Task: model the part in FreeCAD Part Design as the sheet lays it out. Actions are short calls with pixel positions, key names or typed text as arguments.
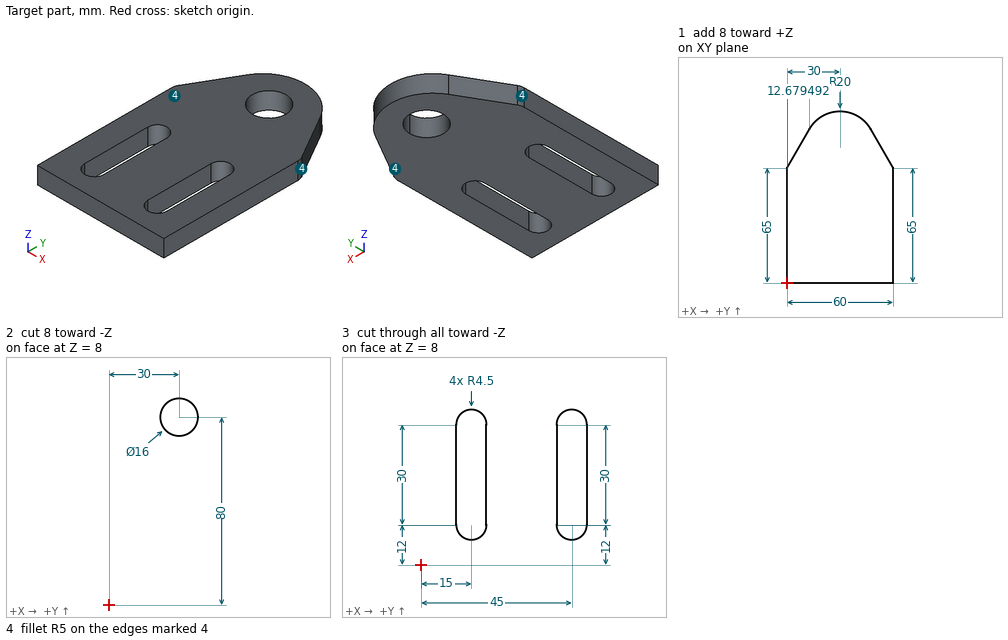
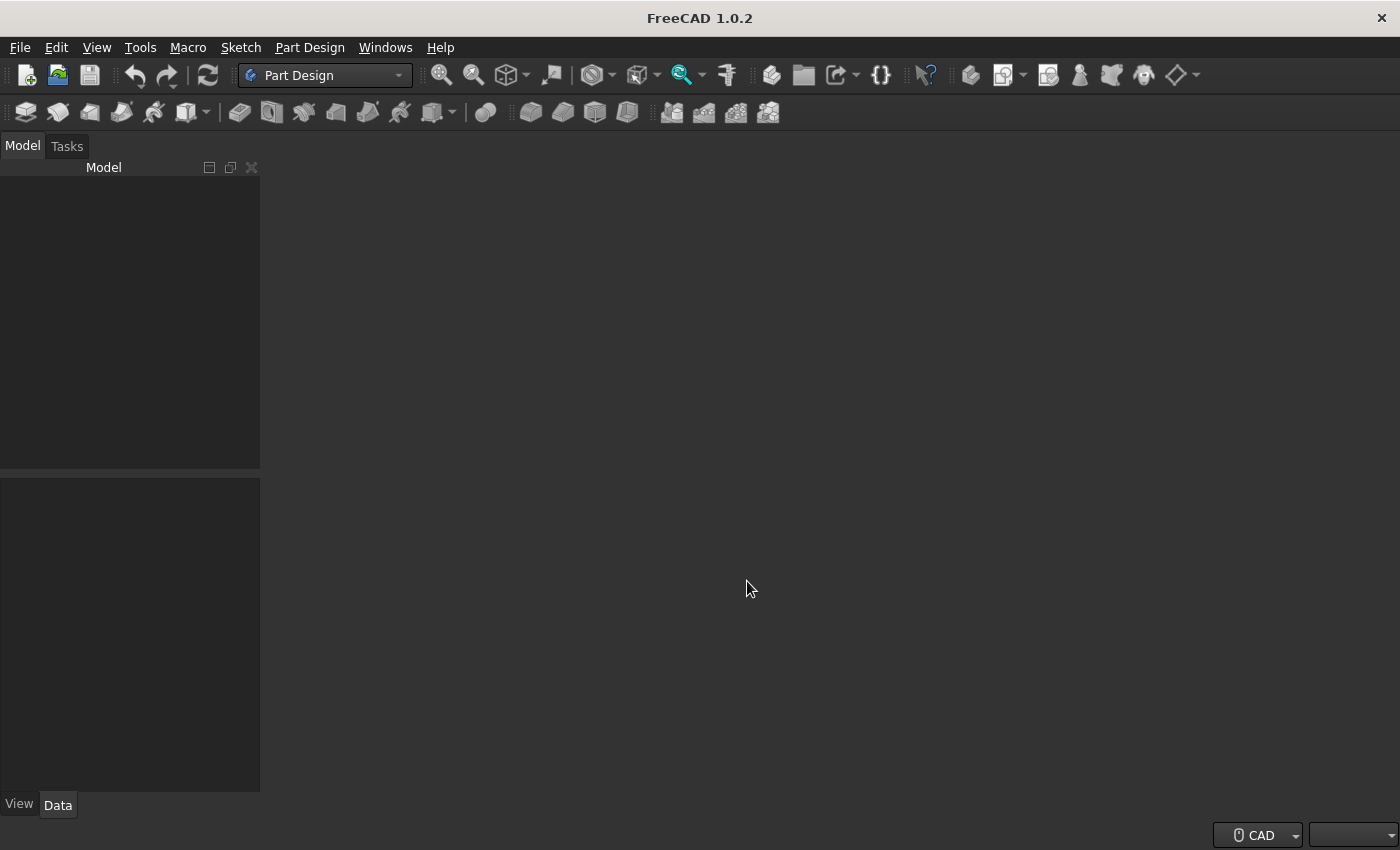
key(ctrl+n)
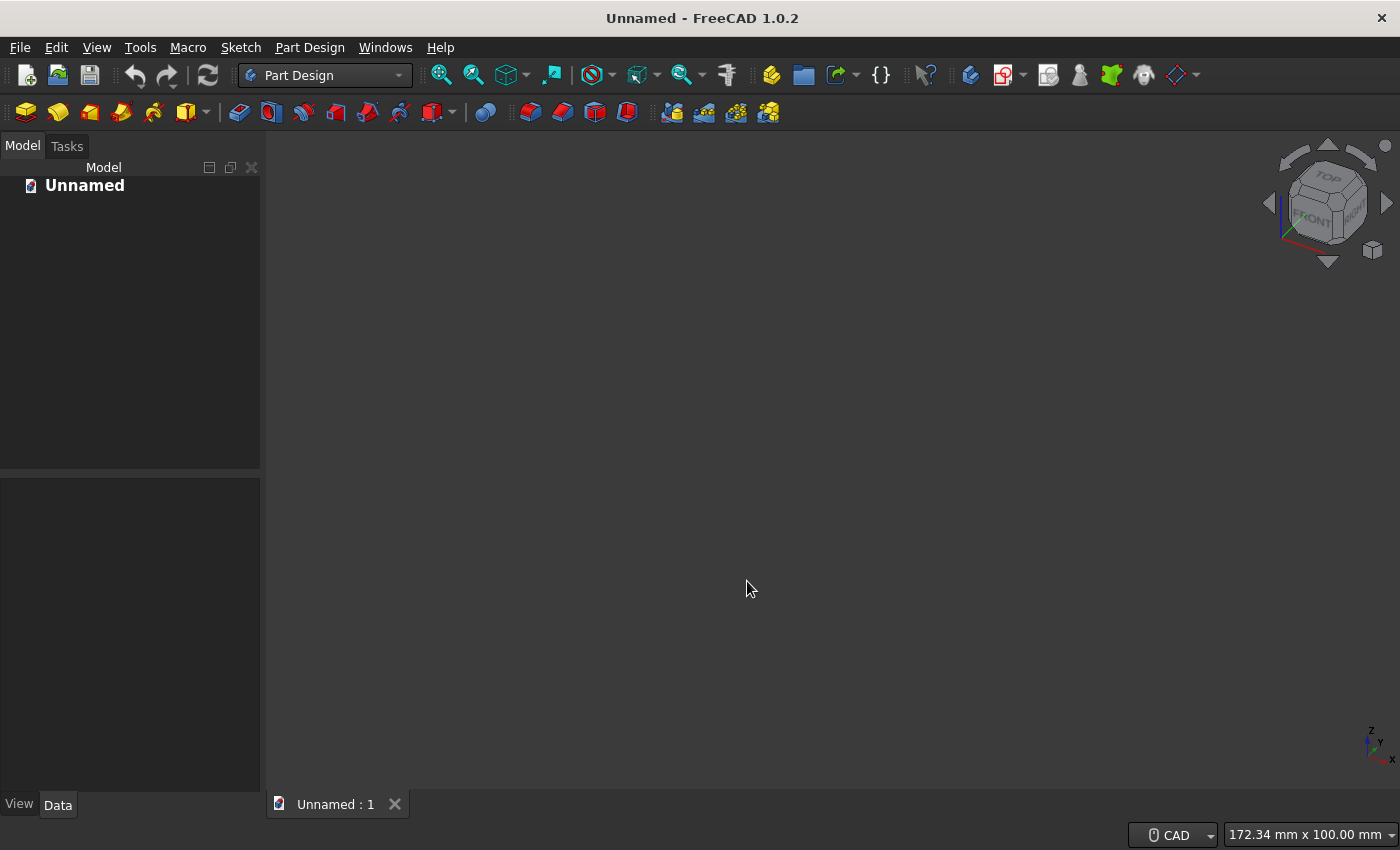
click(1004, 76)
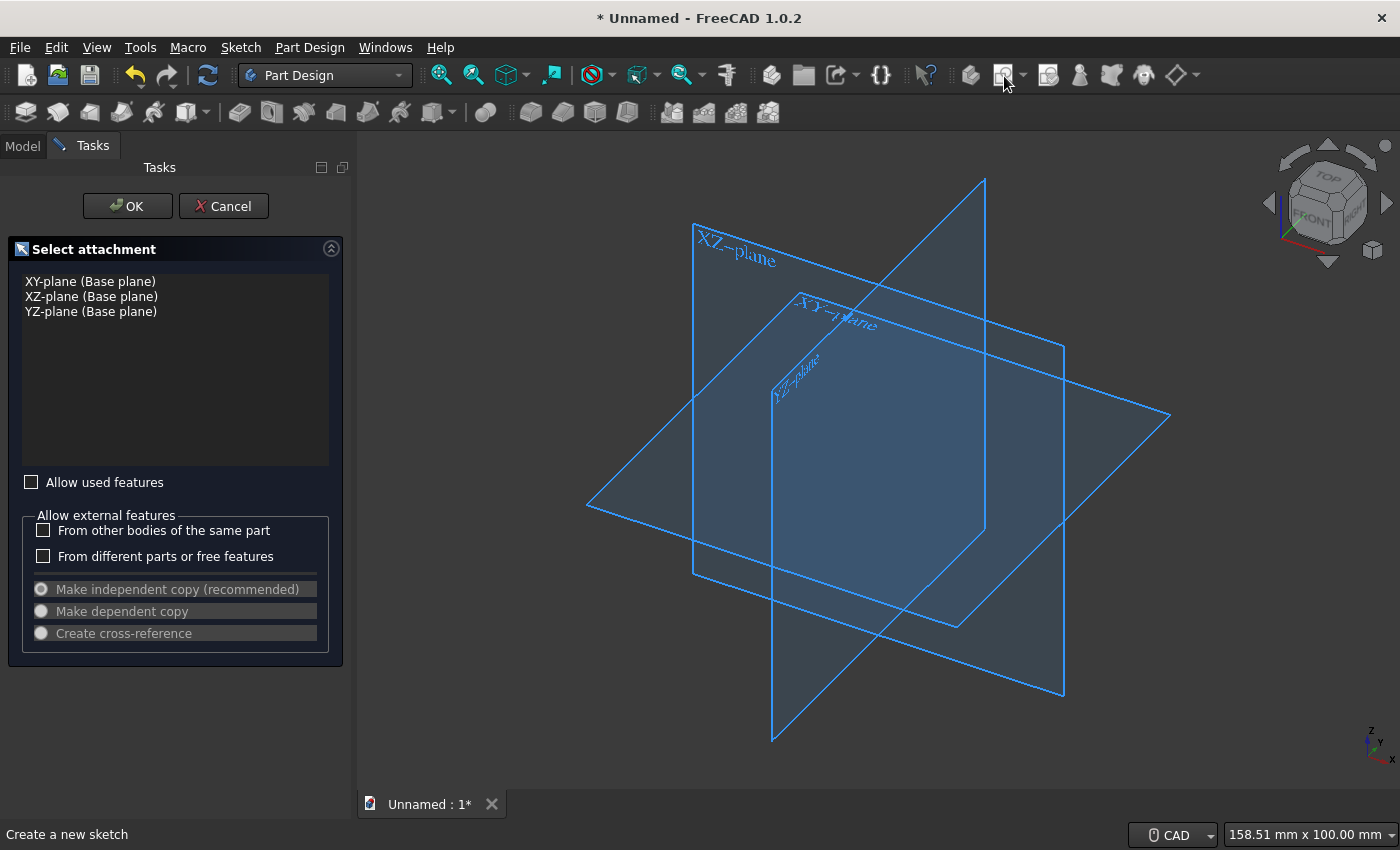
click(82, 282)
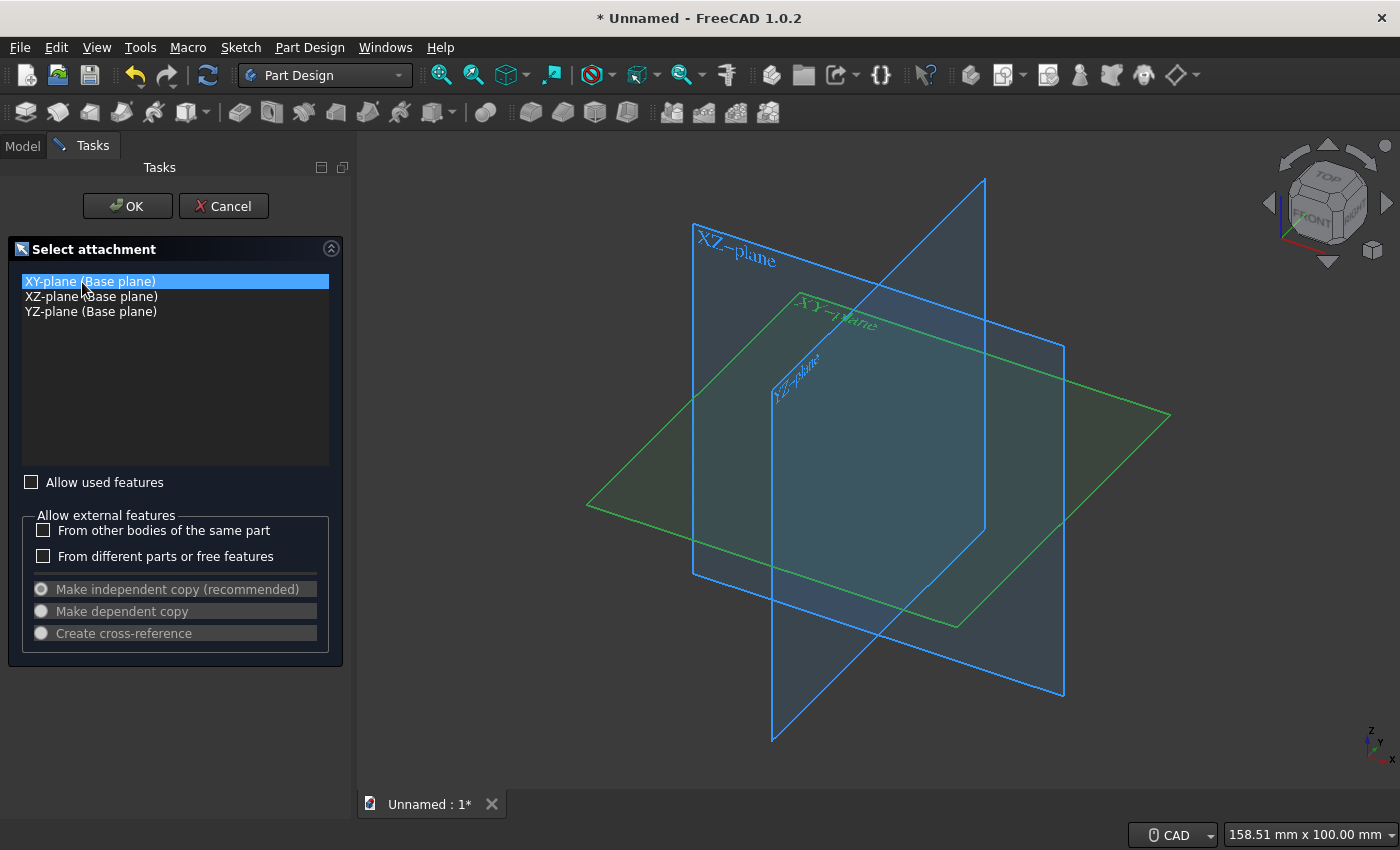
click(128, 206)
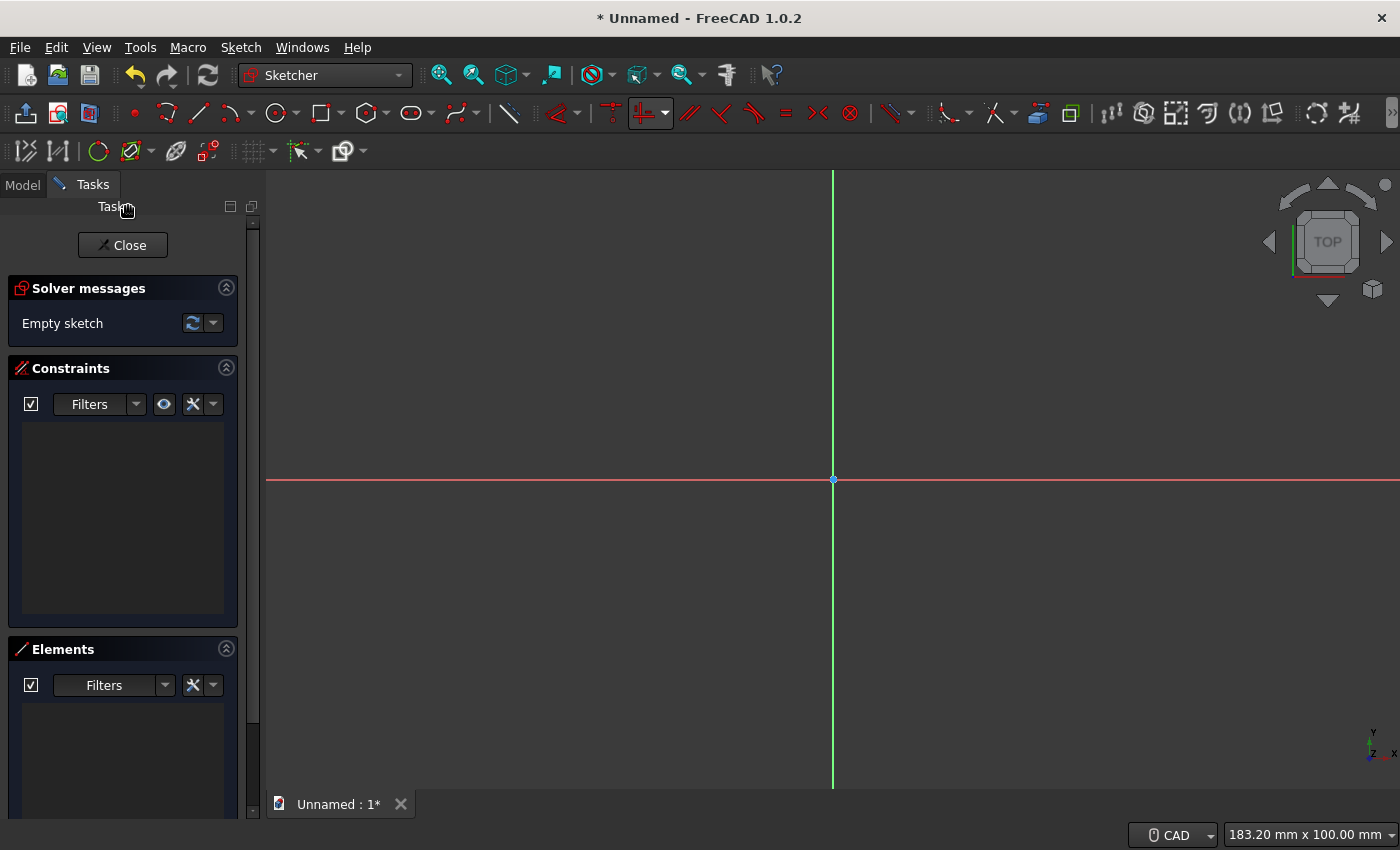
scroll(455, 761, down, 3)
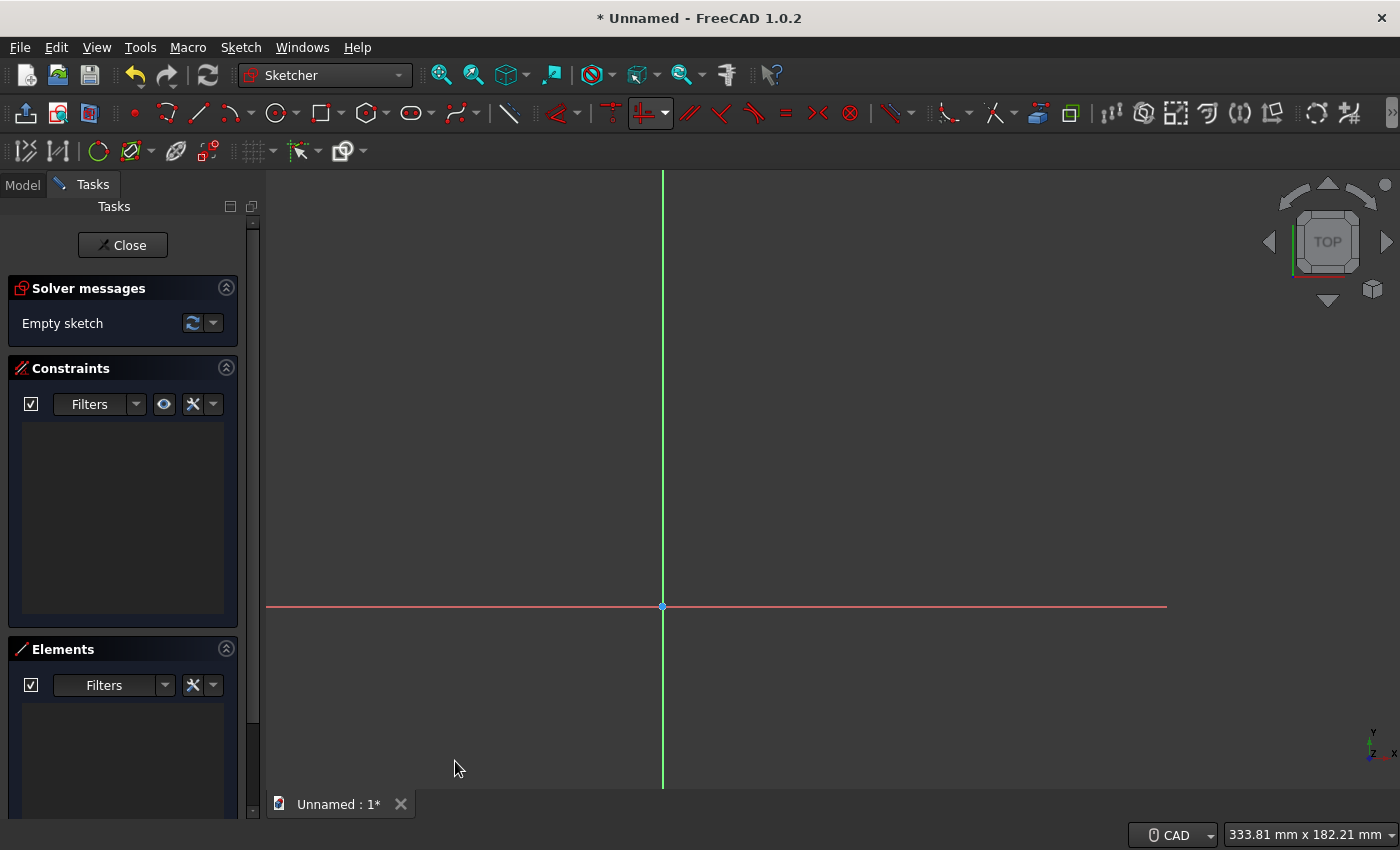
key(g)
key(m)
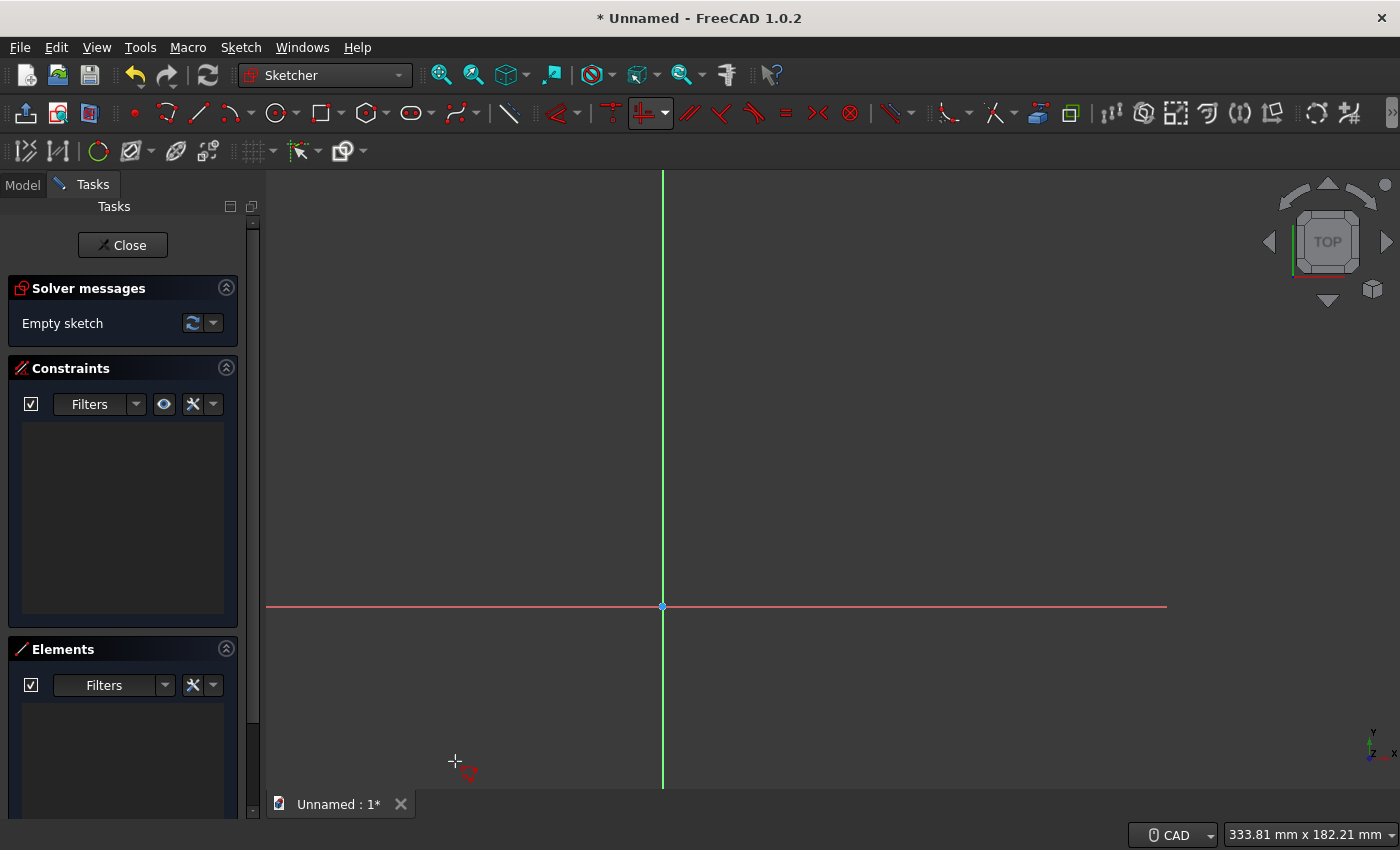
click(706, 312)
click(663, 386)
click(663, 607)
click(866, 598)
click(866, 386)
click(823, 312)
right_click(823, 312)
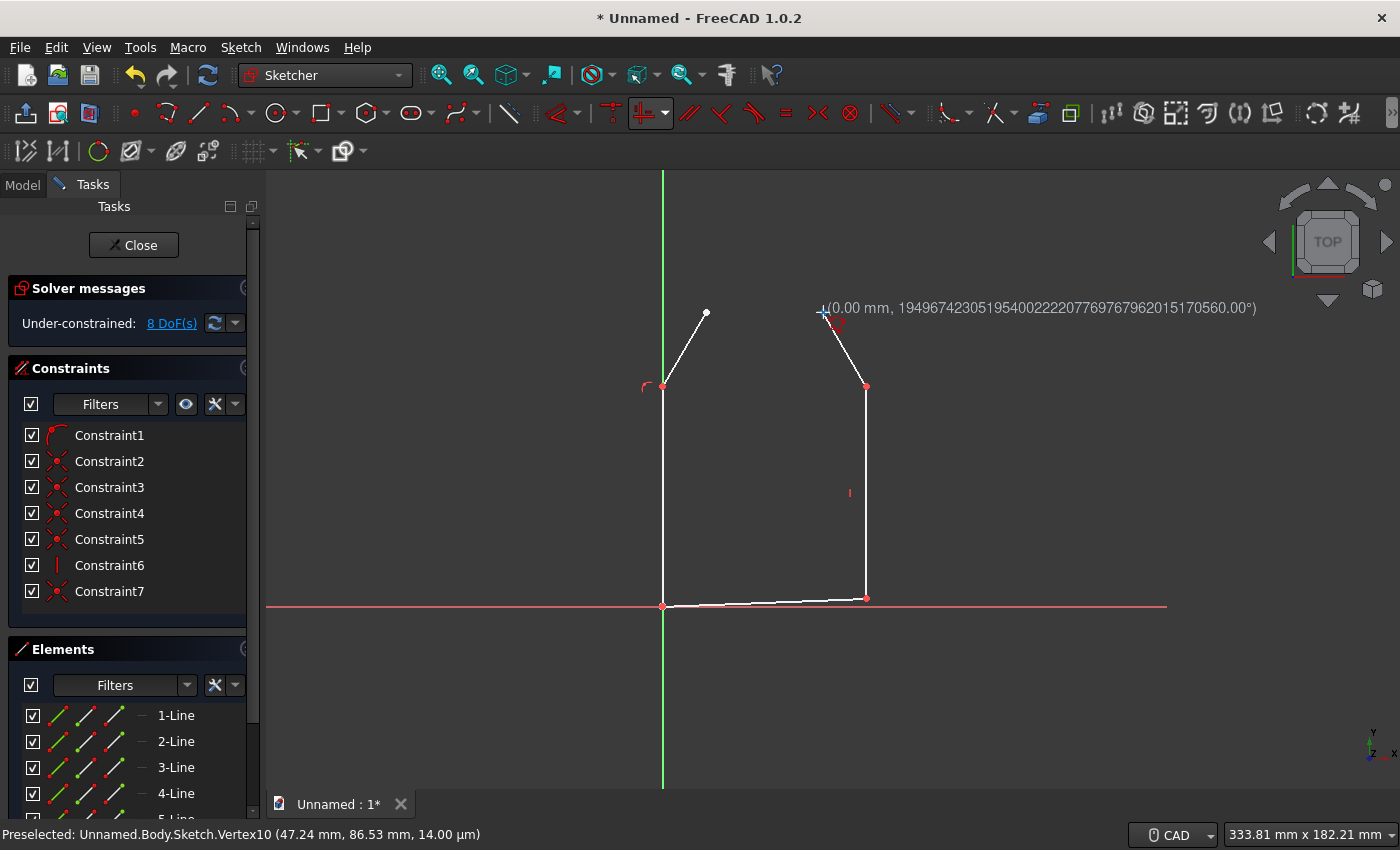
key(g)
key(3)
key(a)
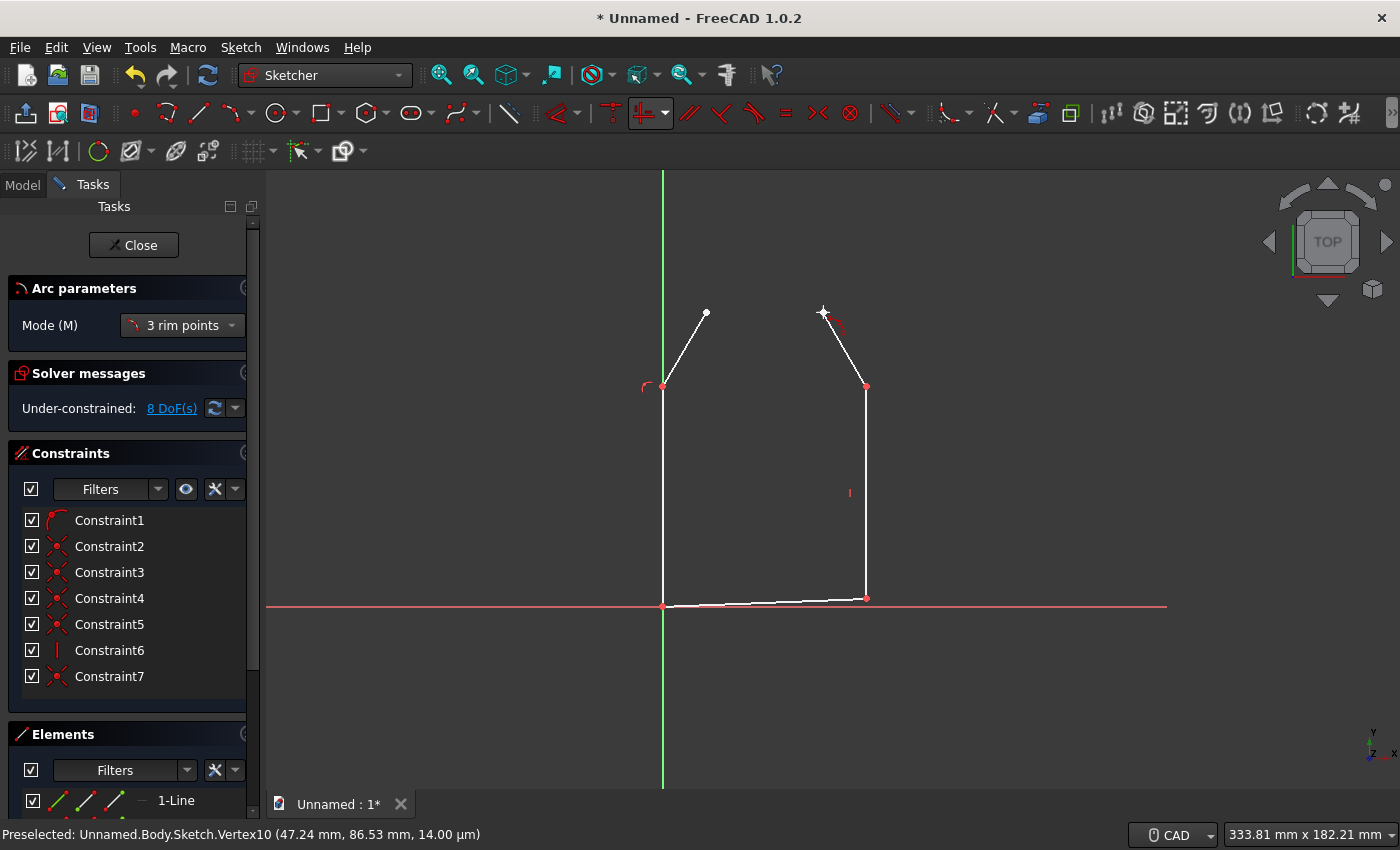
click(823, 313)
click(706, 313)
click(764, 278)
key(Escape)